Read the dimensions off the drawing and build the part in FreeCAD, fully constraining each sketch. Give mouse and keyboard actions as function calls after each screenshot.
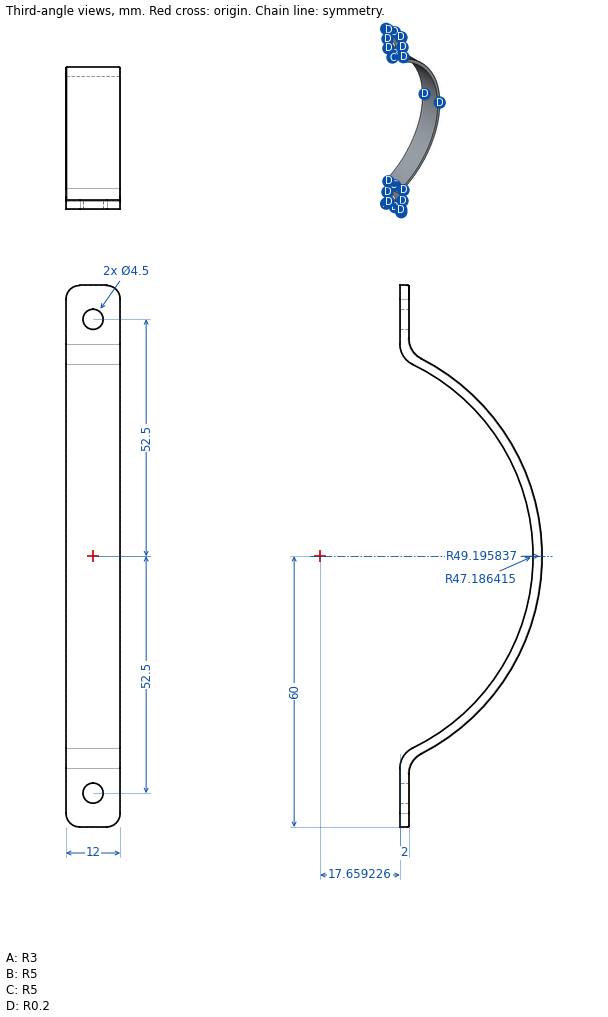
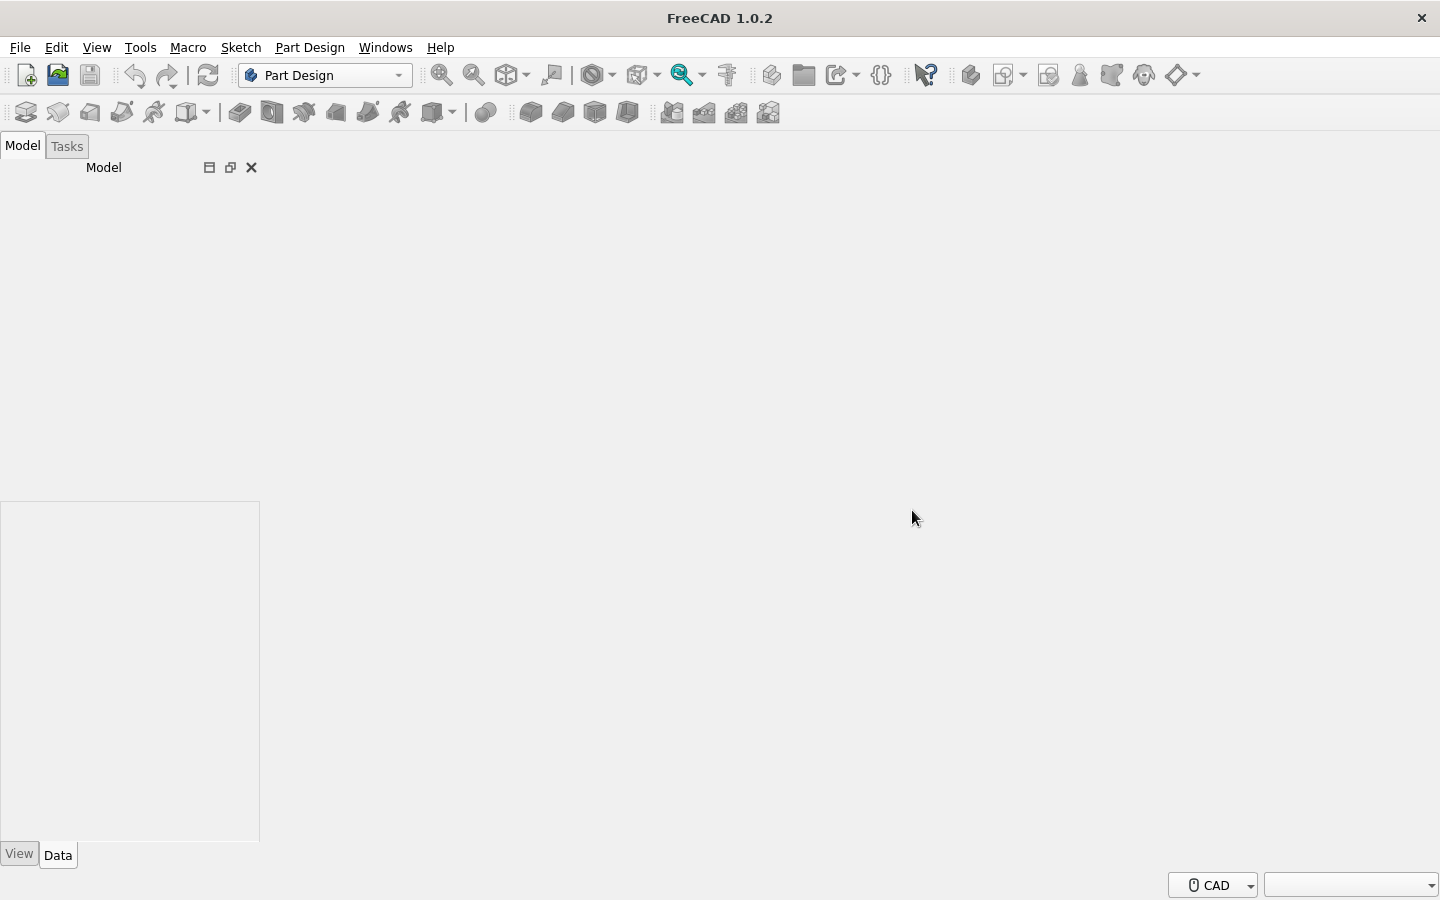
click(26, 76)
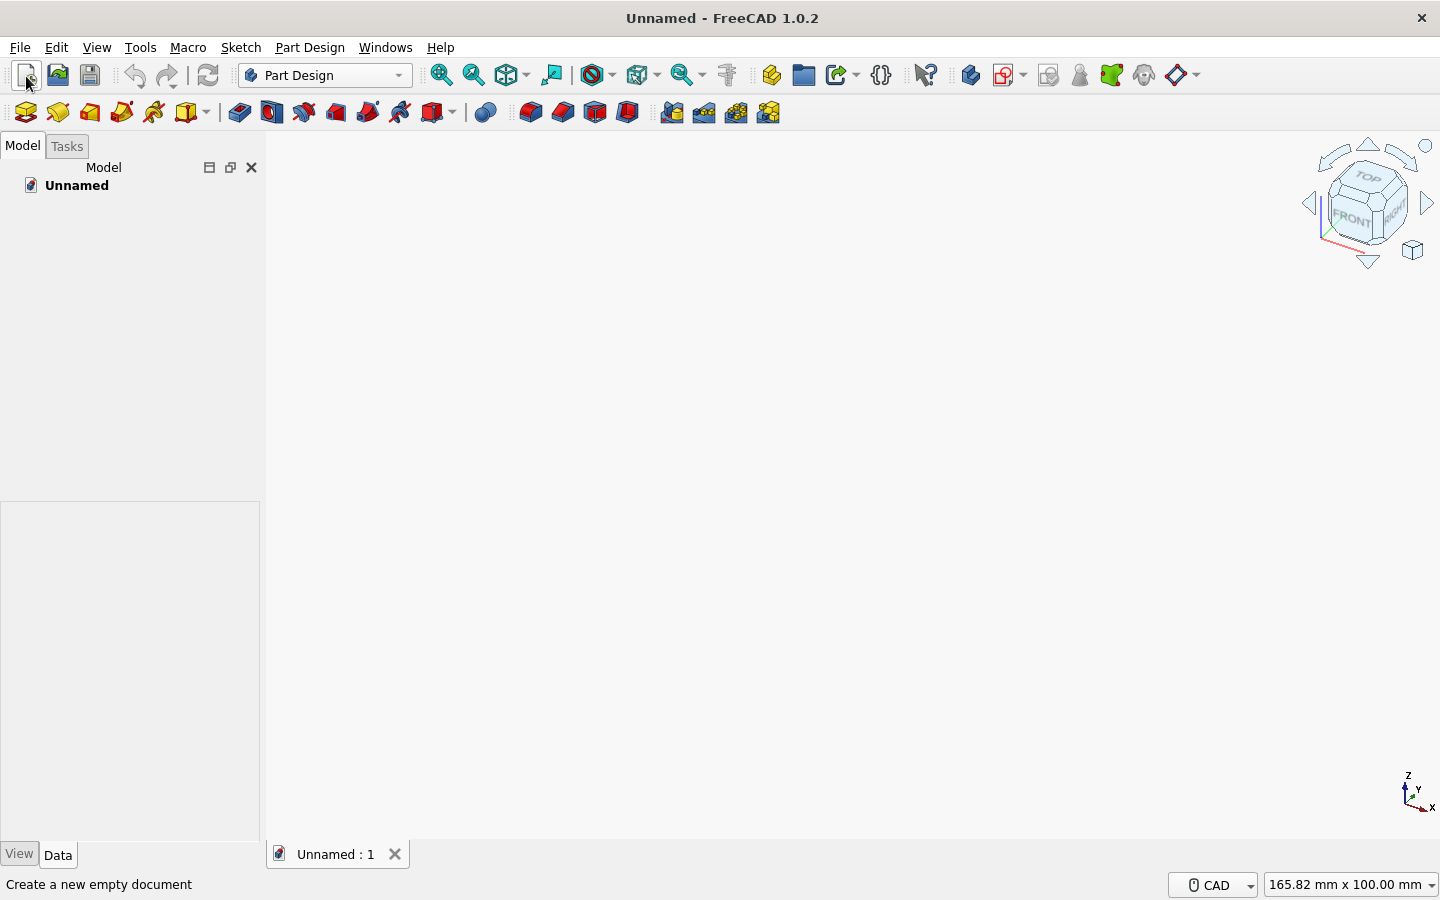
click(1004, 76)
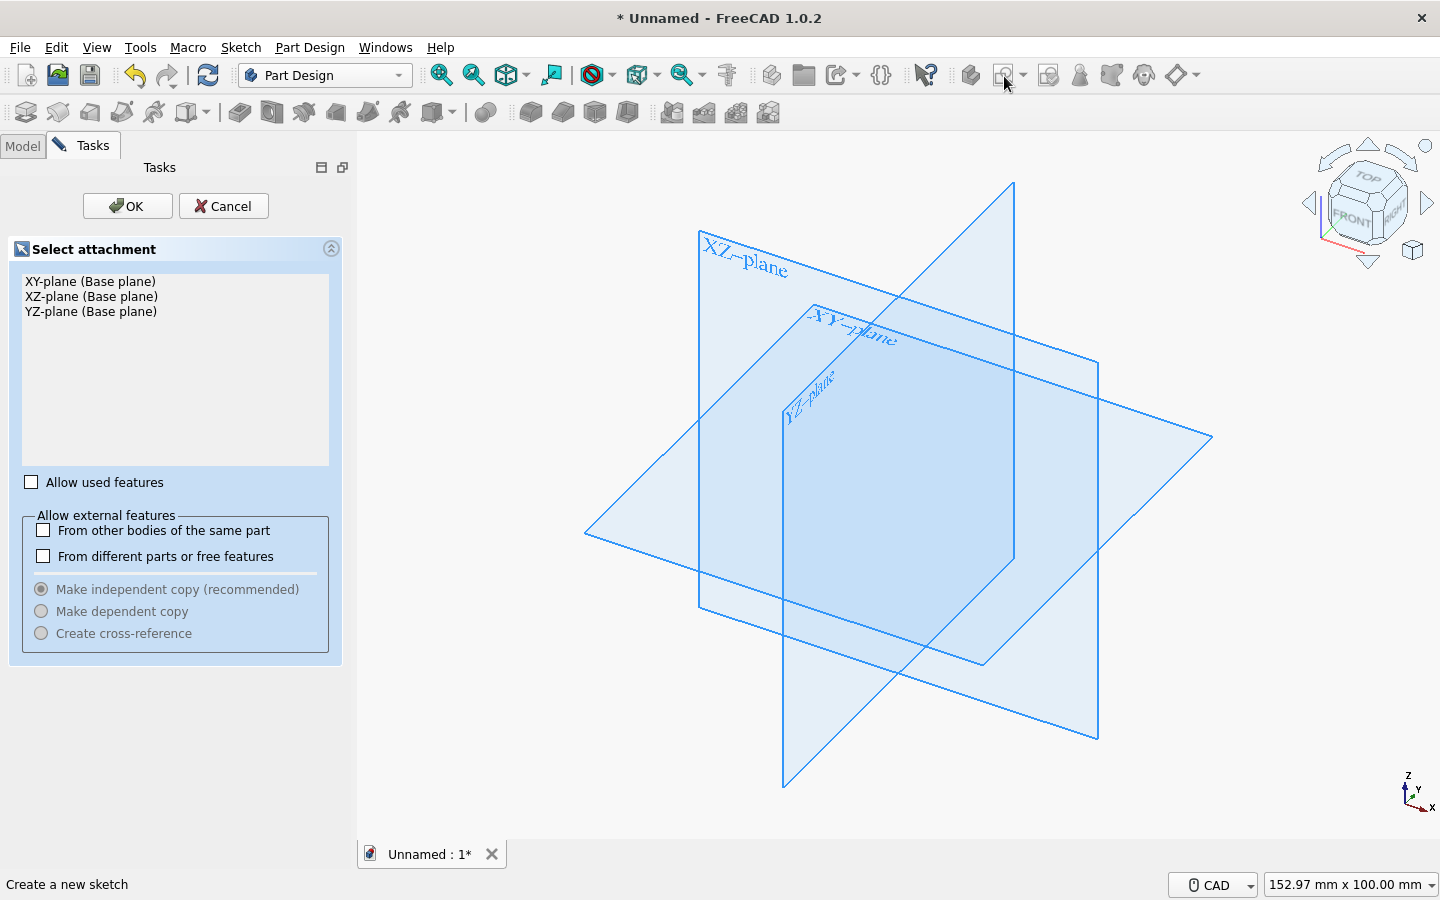
click(82, 312)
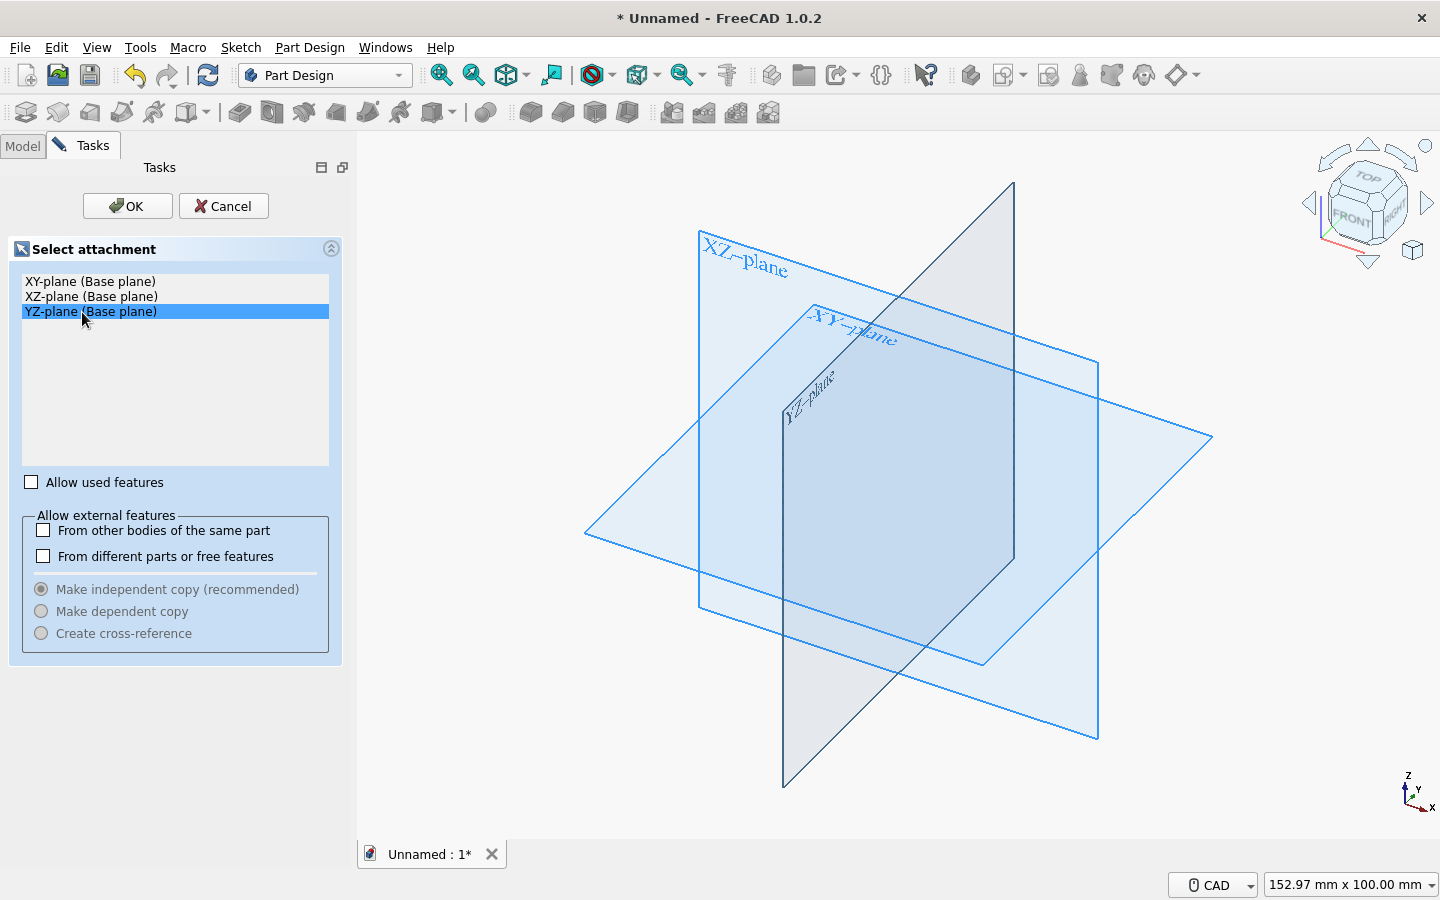
click(128, 206)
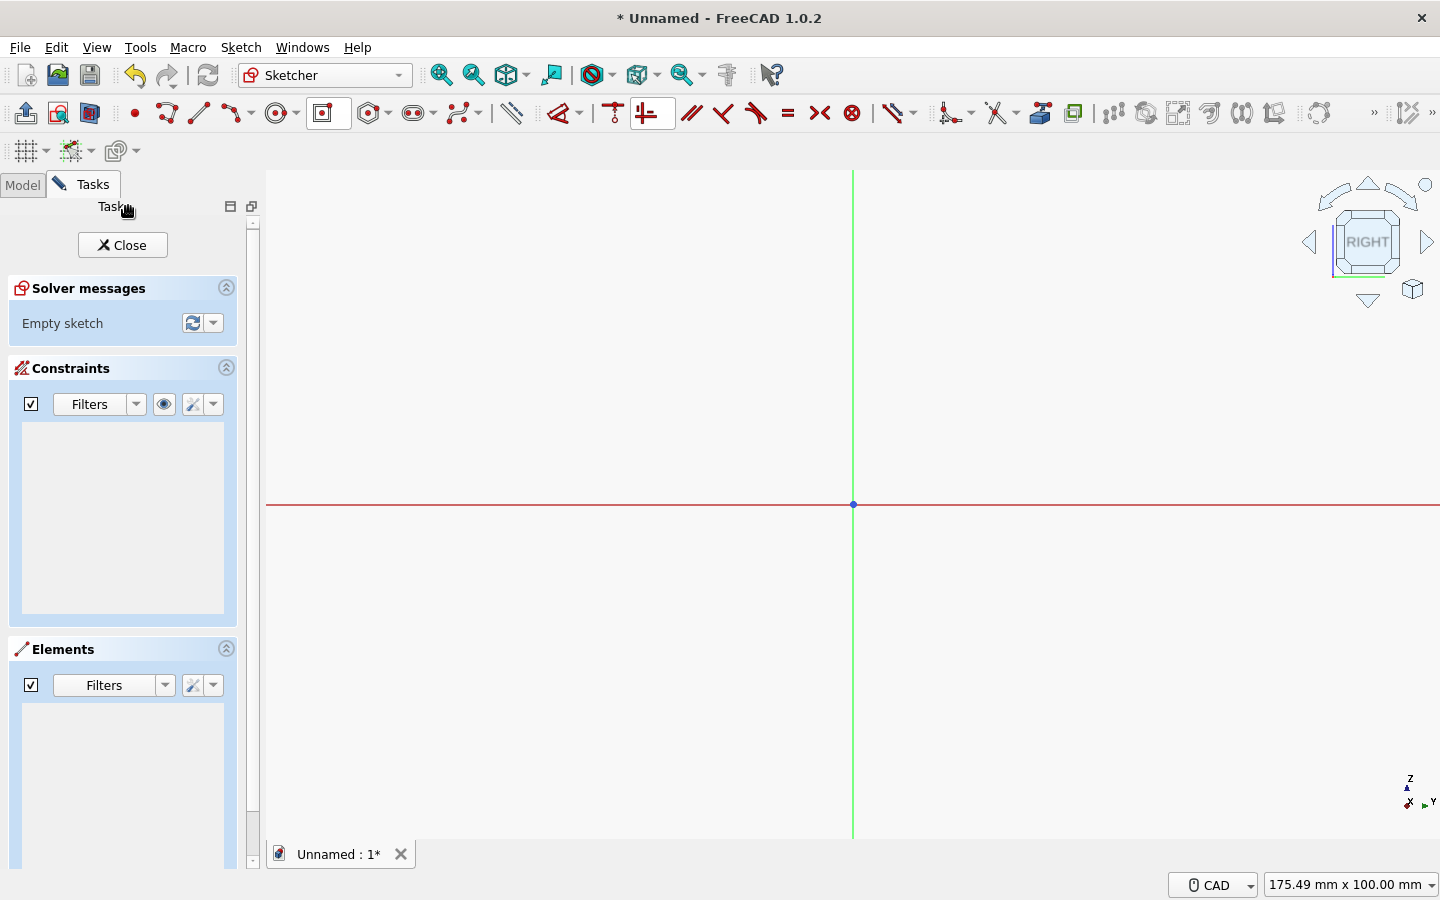
scroll(501, 504, down, 3)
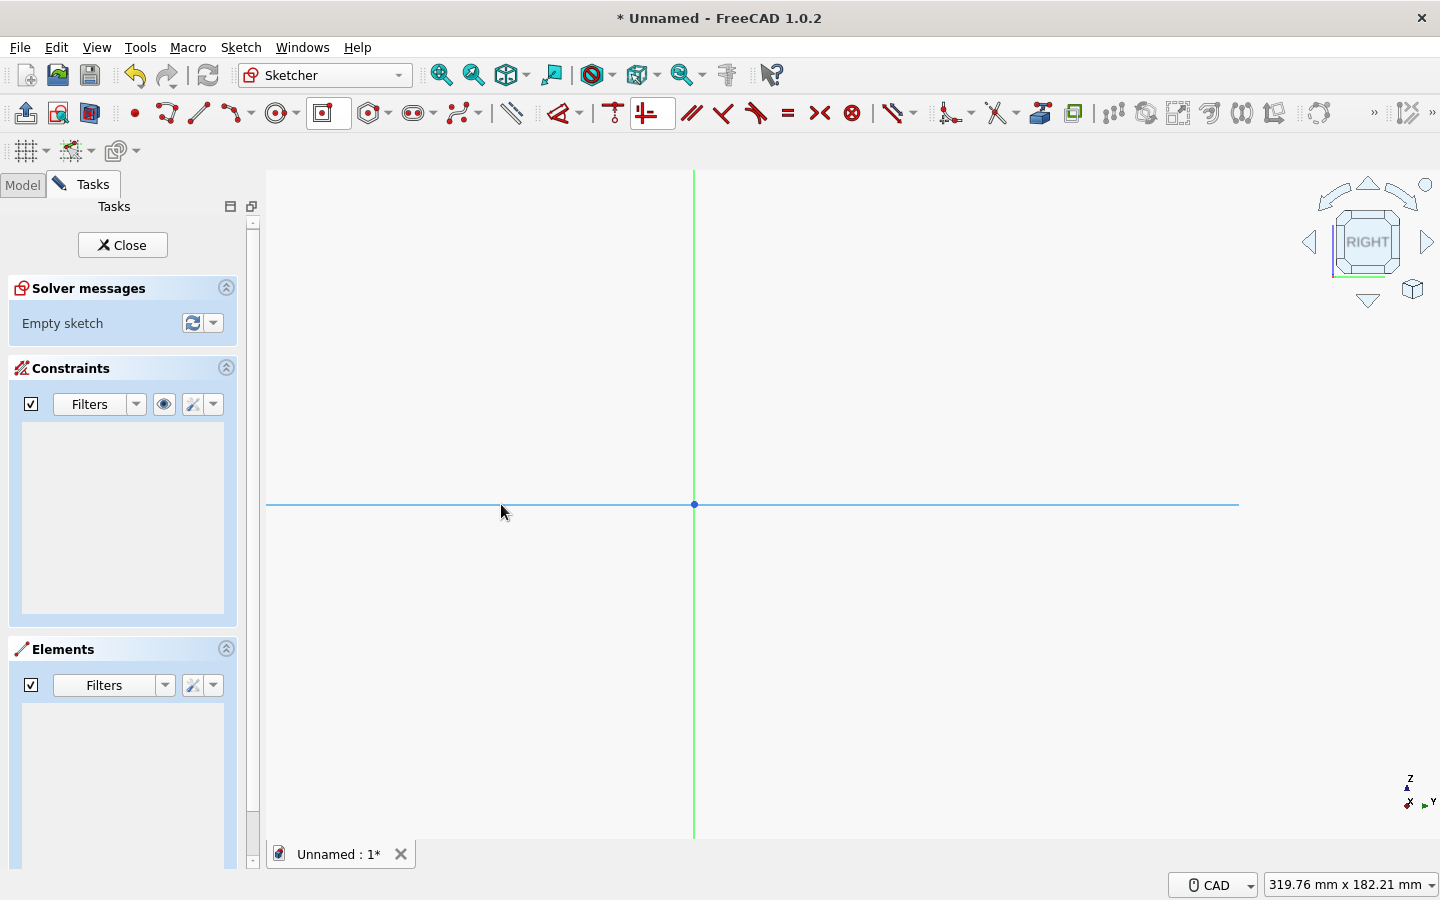
click(168, 114)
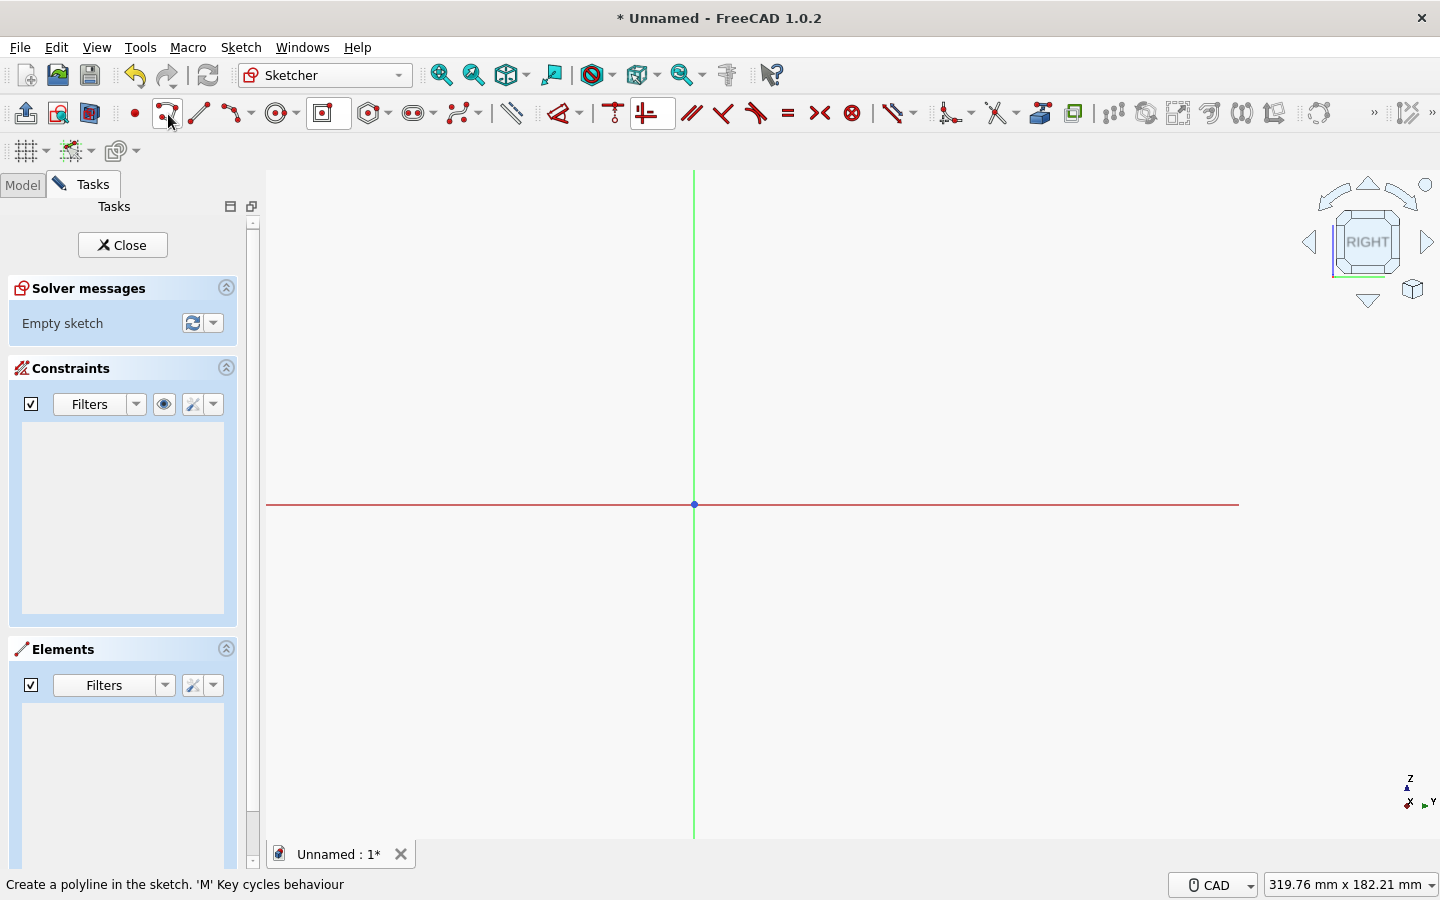
click(759, 665)
click(759, 725)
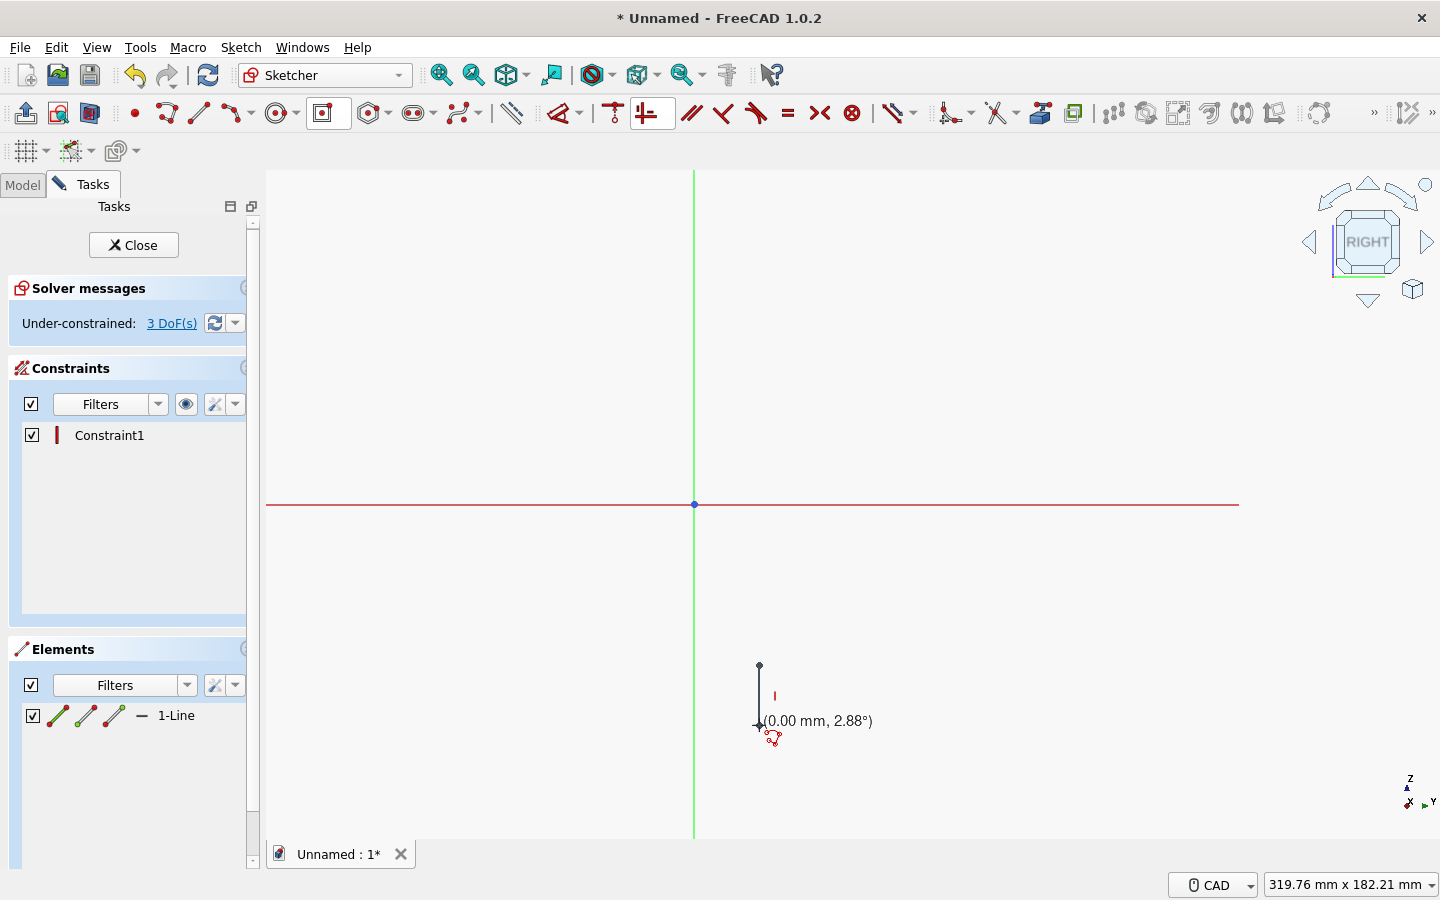
scroll(766, 725, up, 4)